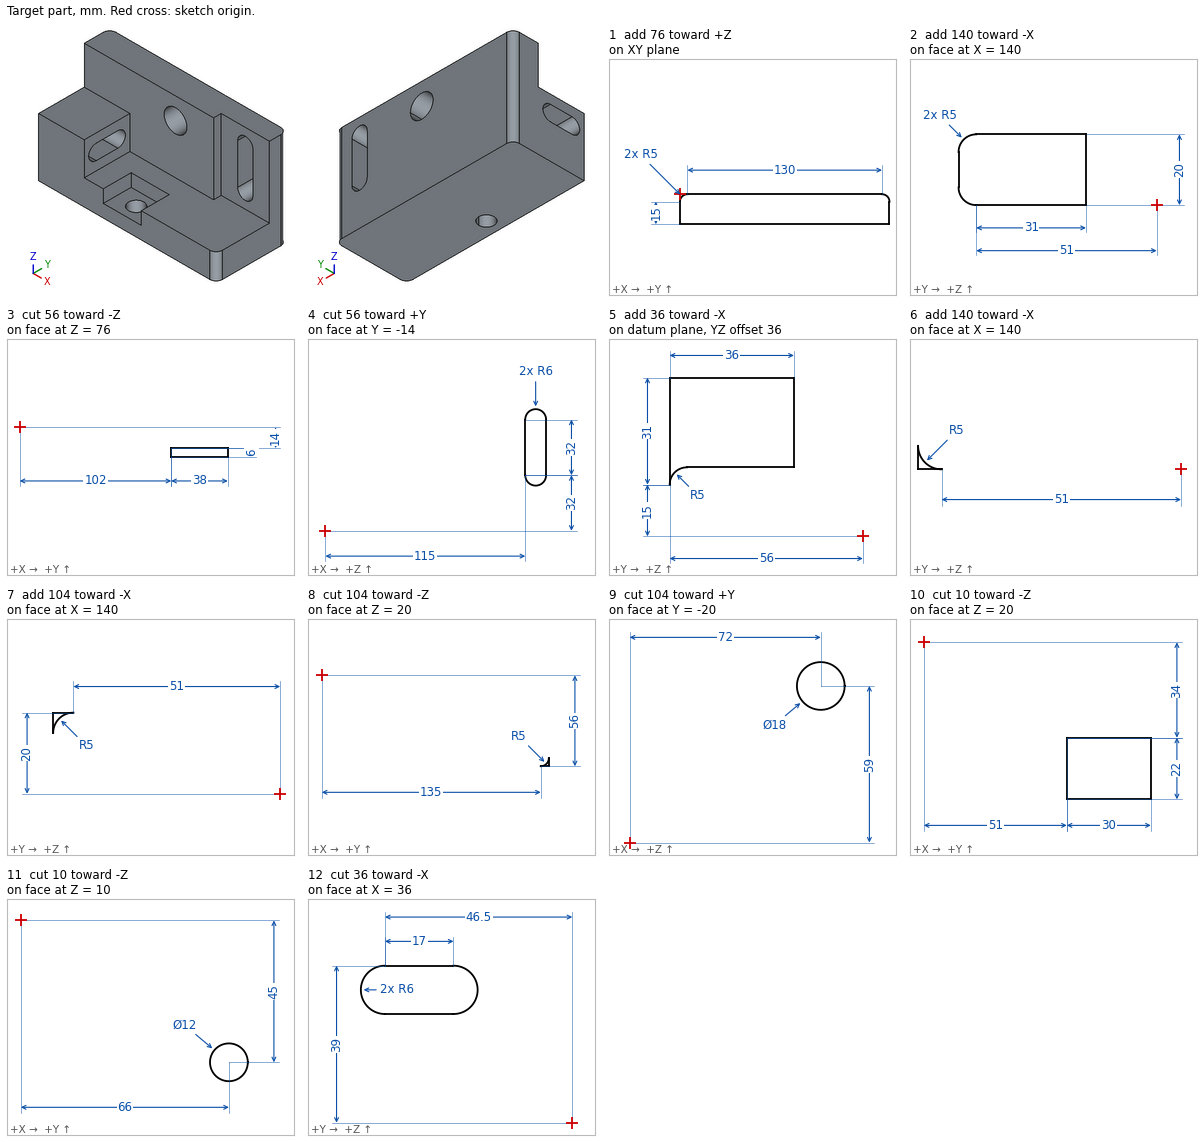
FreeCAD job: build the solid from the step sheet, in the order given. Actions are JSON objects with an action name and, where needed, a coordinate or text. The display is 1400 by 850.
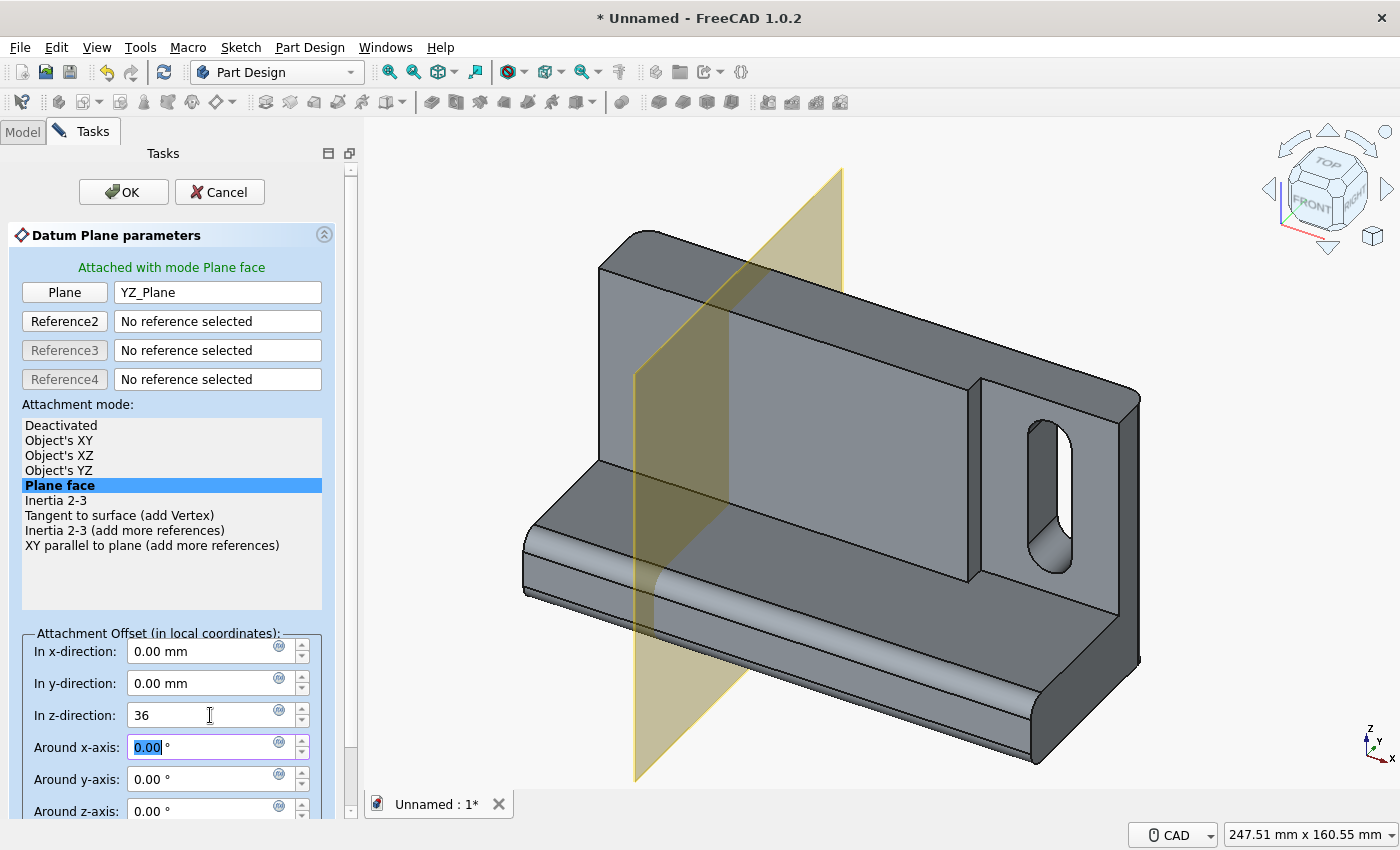
{"action": "left_click", "coordinate": [124, 192]}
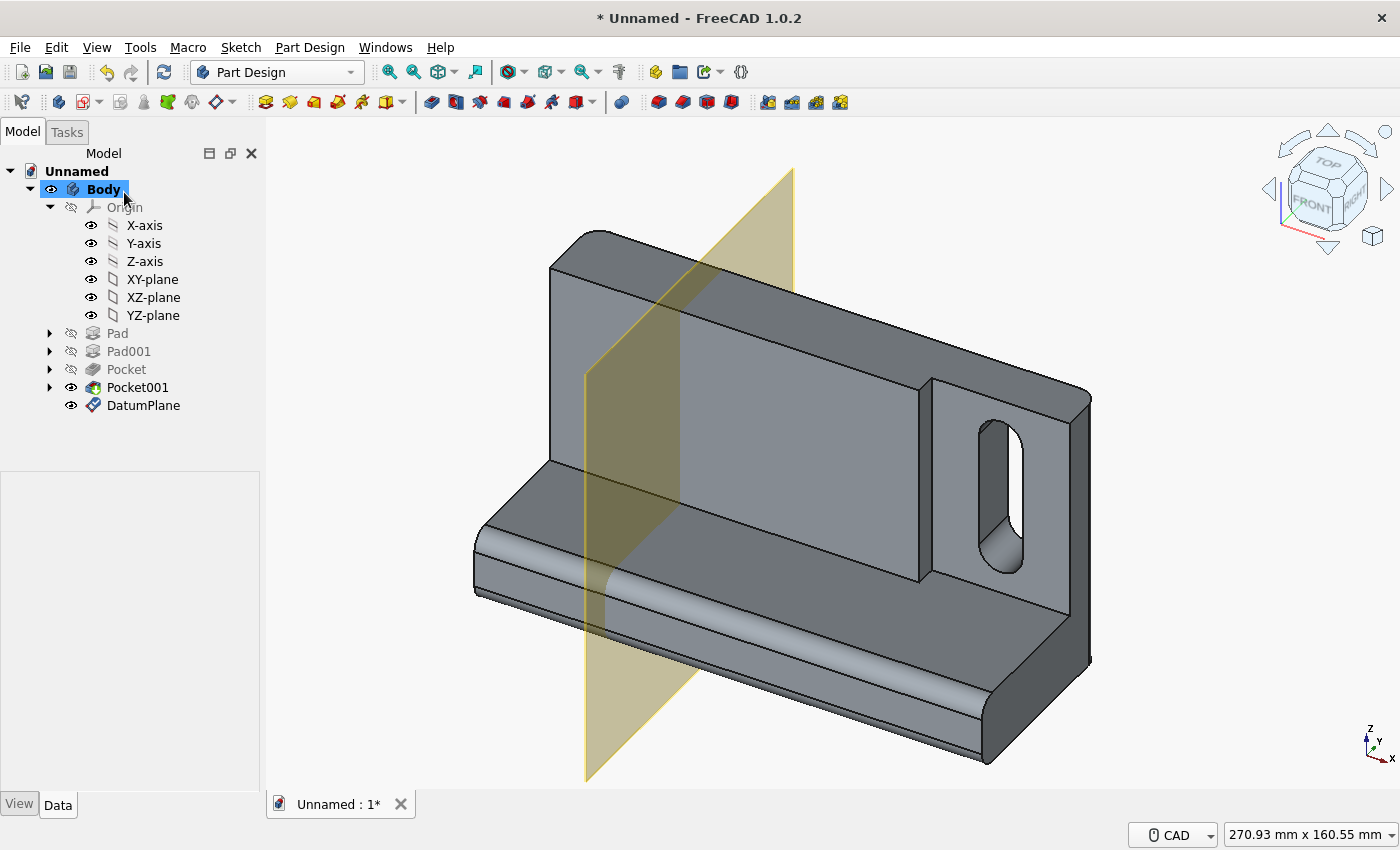
{"action": "left_click", "coordinate": [116, 405]}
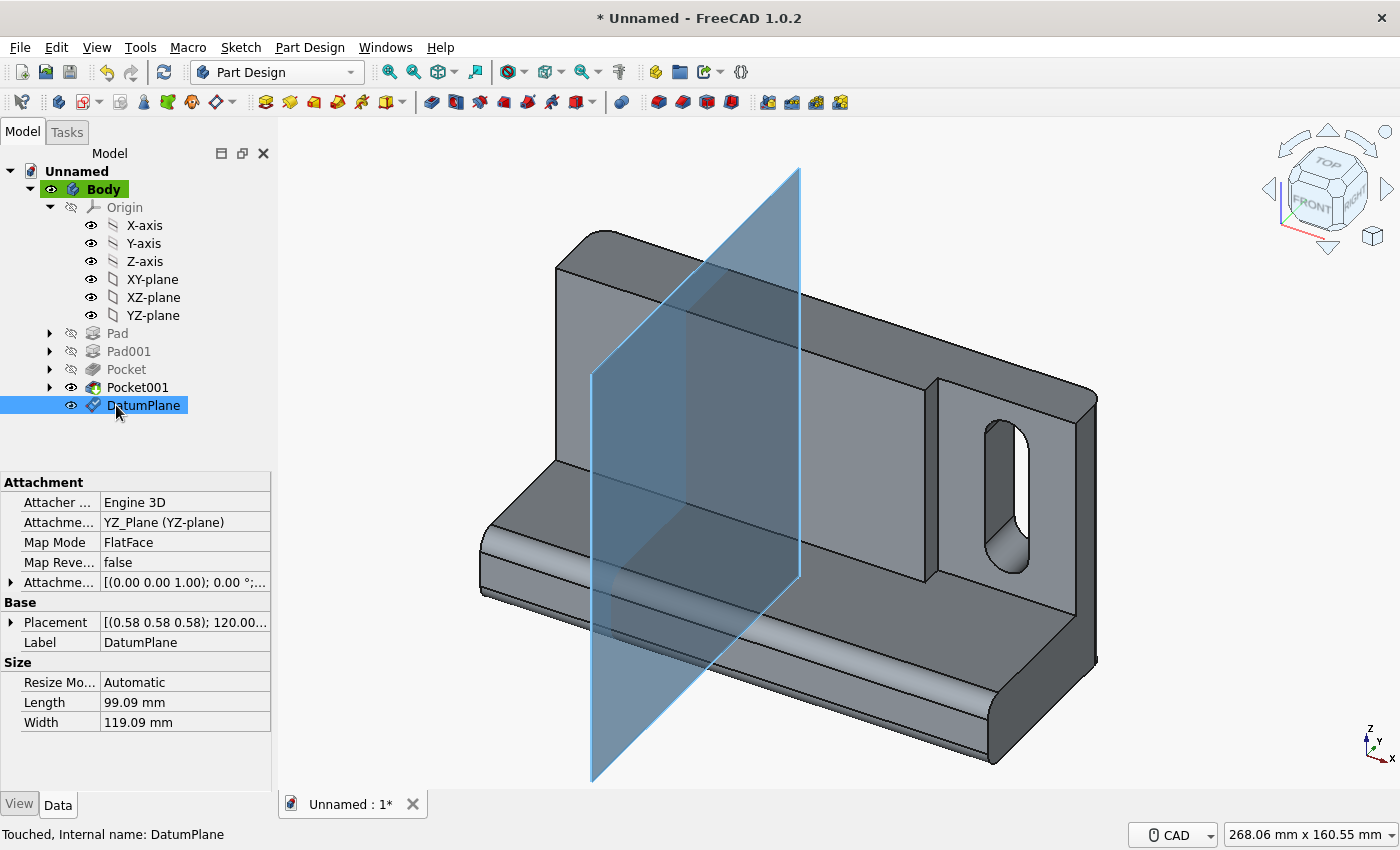
{"action": "left_click", "coordinate": [84, 102]}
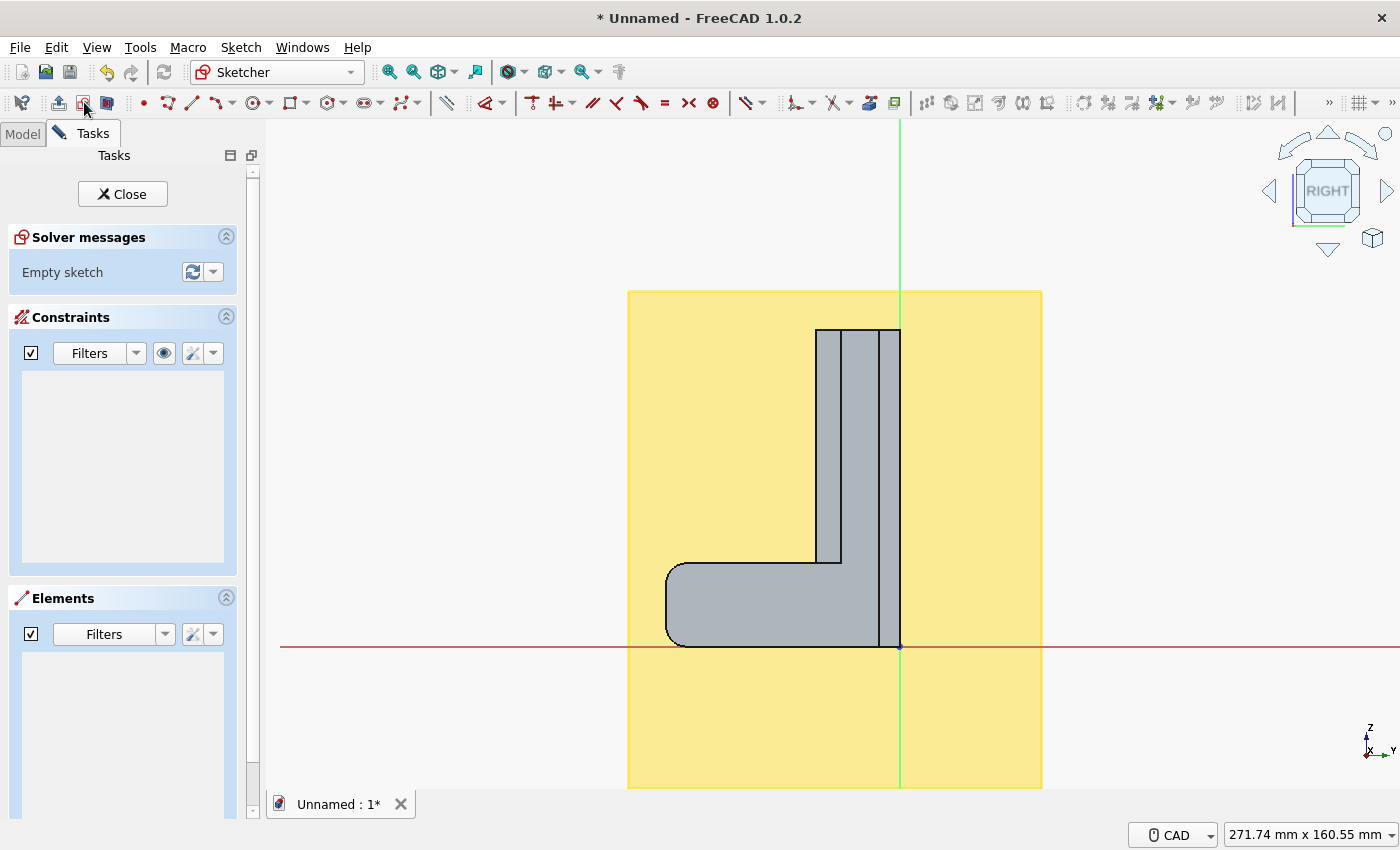
{"action": "left_click", "coordinate": [108, 104]}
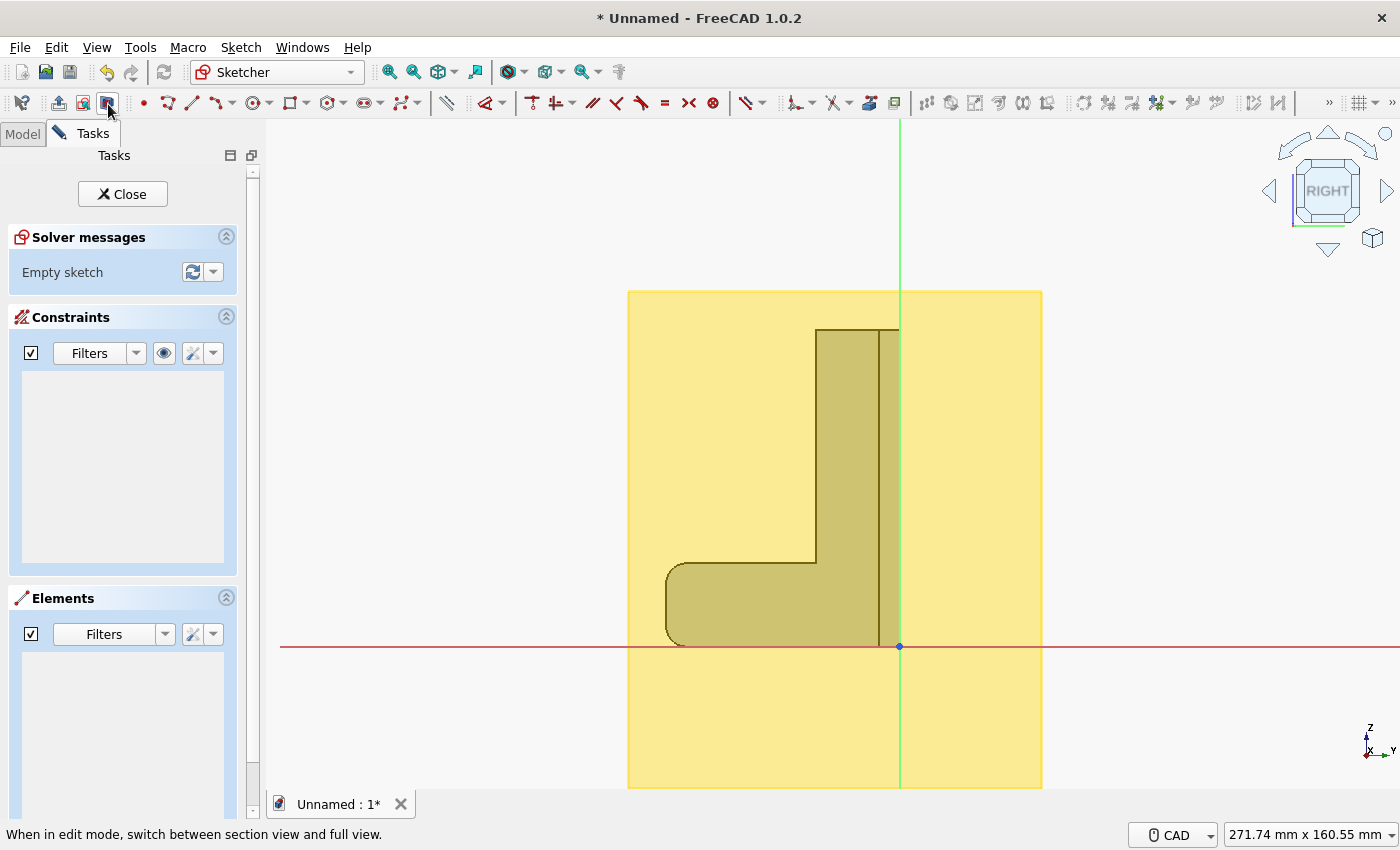
{"action": "scroll", "coordinate": [798, 630], "scroll_direction": "up", "scroll_amount": 4}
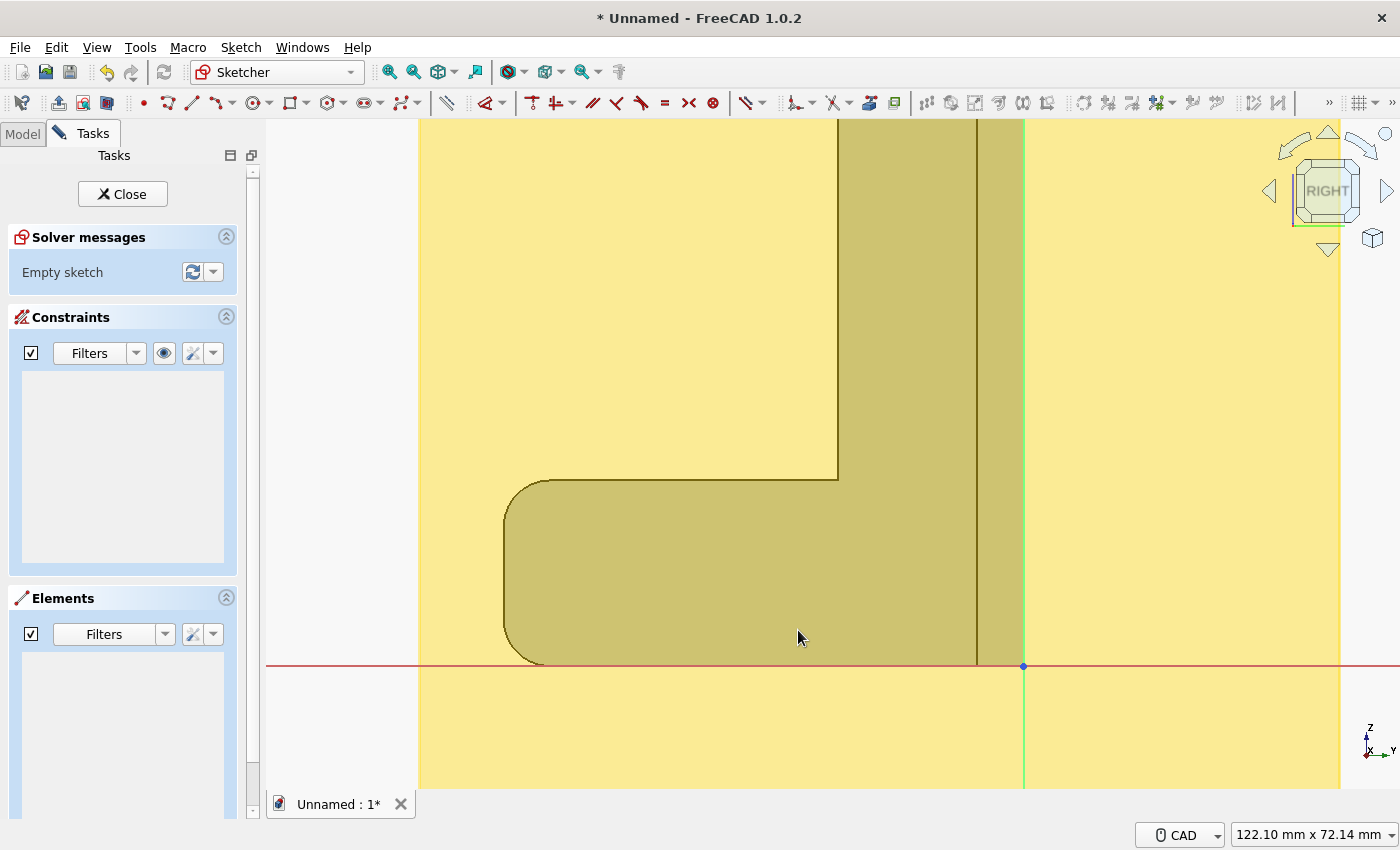
{"action": "left_click", "coordinate": [168, 104]}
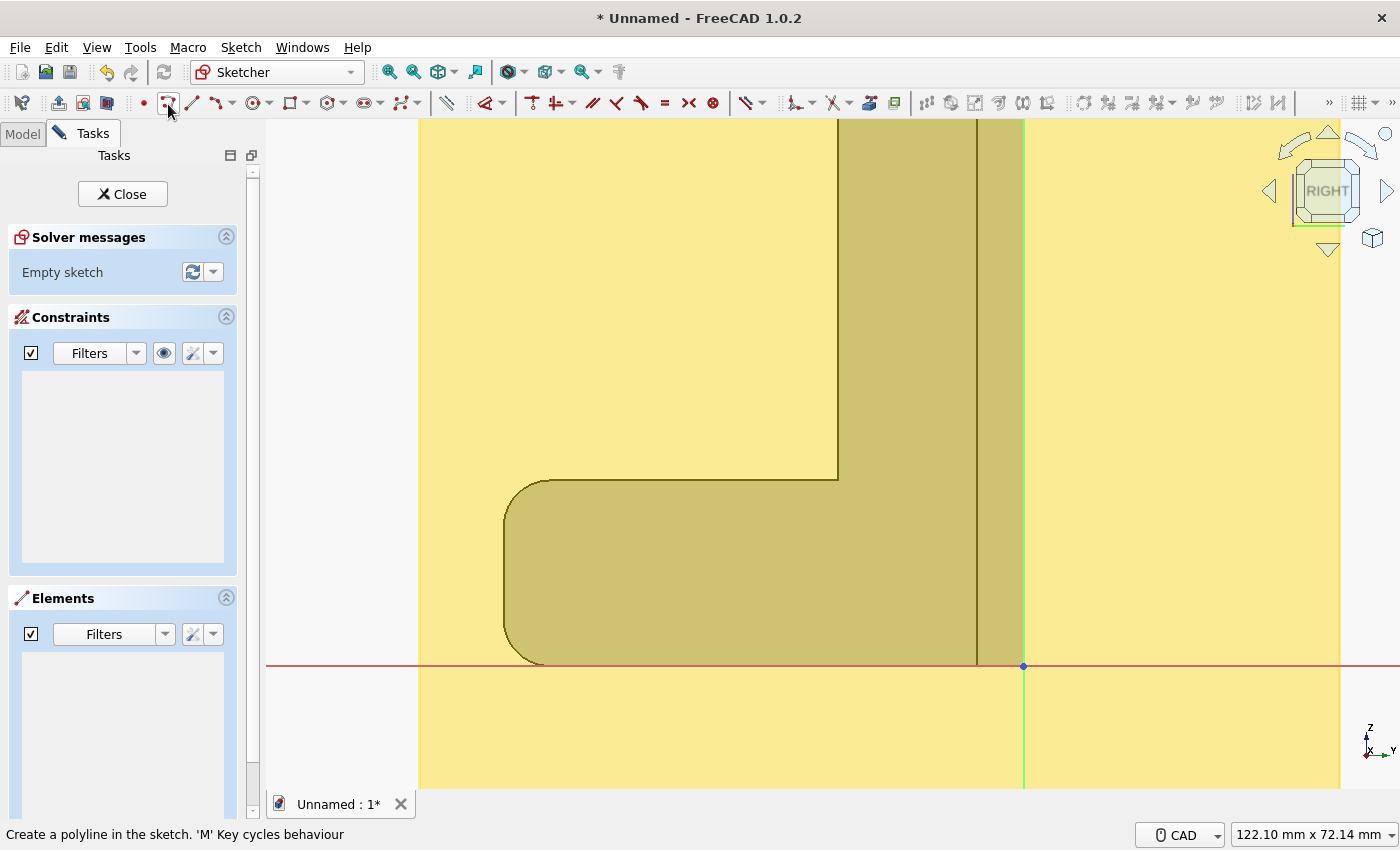
{"action": "left_click", "coordinate": [504, 527]}
{"action": "left_click", "coordinate": [504, 239]}
{"action": "left_click", "coordinate": [838, 239]}
{"action": "left_click", "coordinate": [838, 480]}
{"action": "left_click", "coordinate": [550, 480]}
{"action": "right_click", "coordinate": [550, 480]}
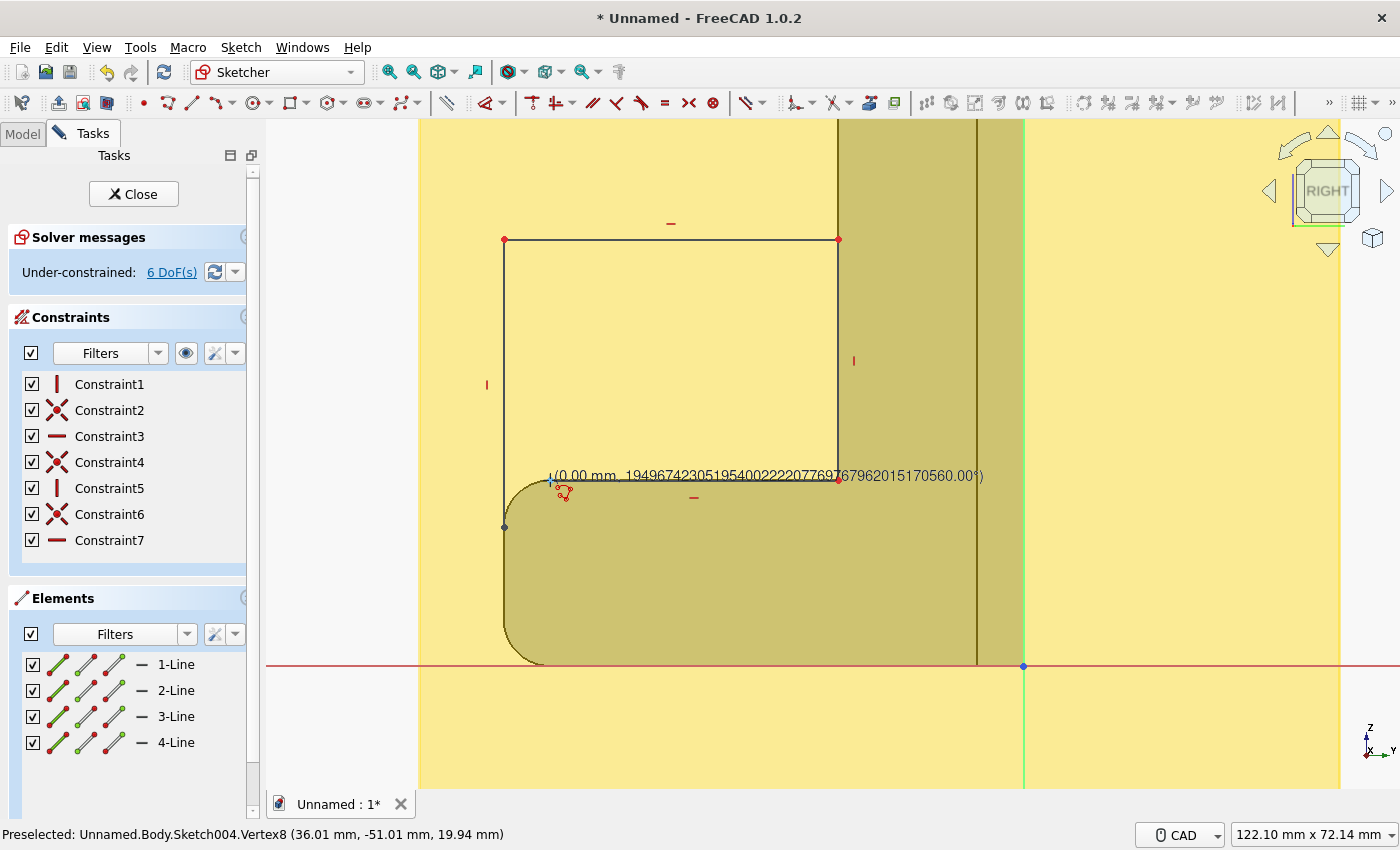
{"action": "left_click", "coordinate": [216, 104]}